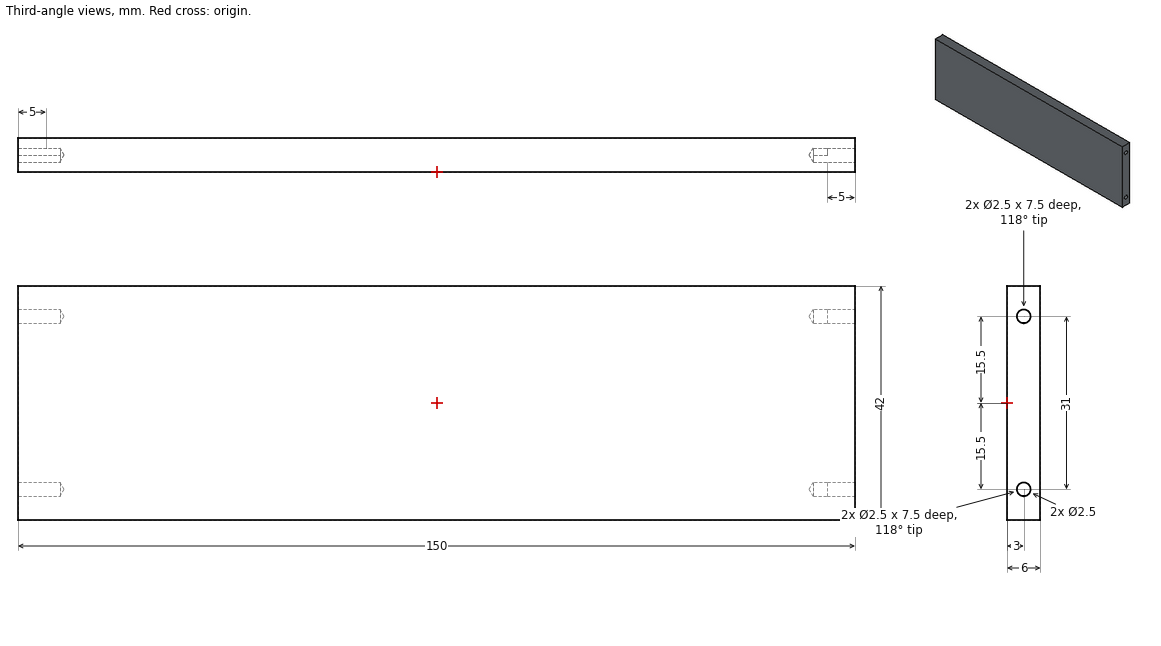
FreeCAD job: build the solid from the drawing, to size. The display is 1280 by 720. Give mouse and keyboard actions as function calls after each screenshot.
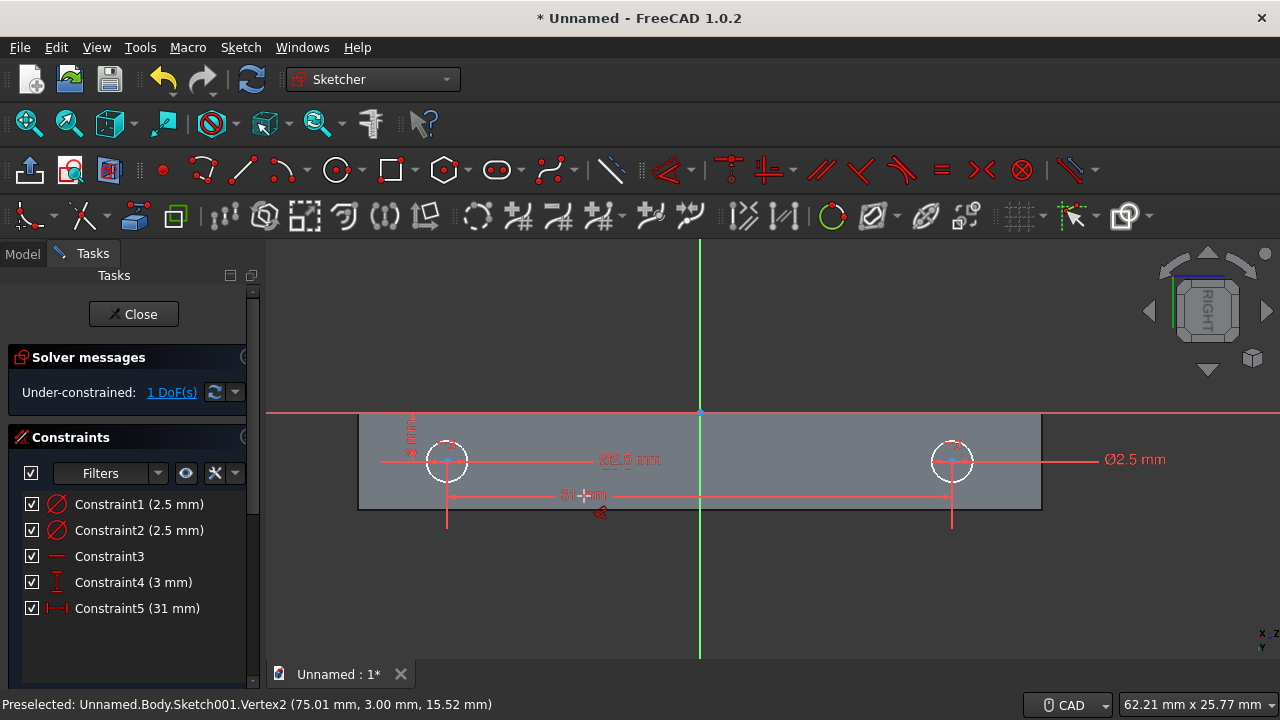
click(447, 462)
click(574, 379)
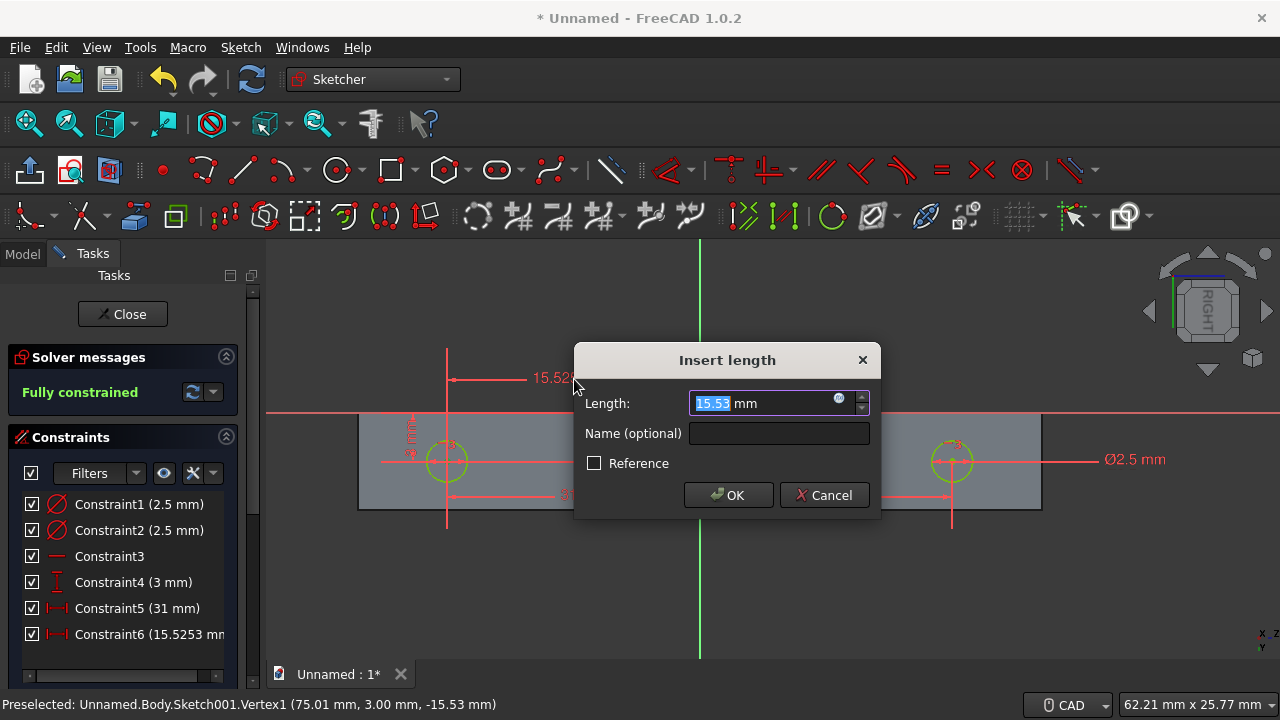
text(15.5)
key(Return)
key(Escape)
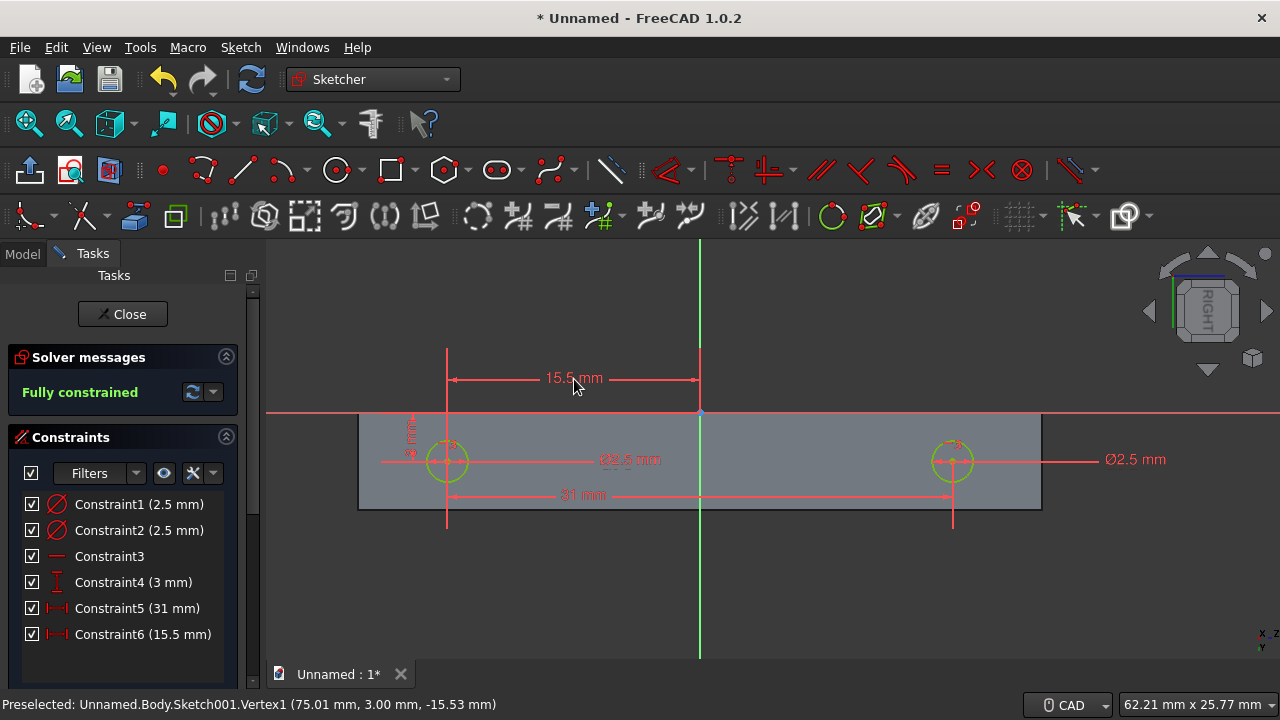
click(123, 314)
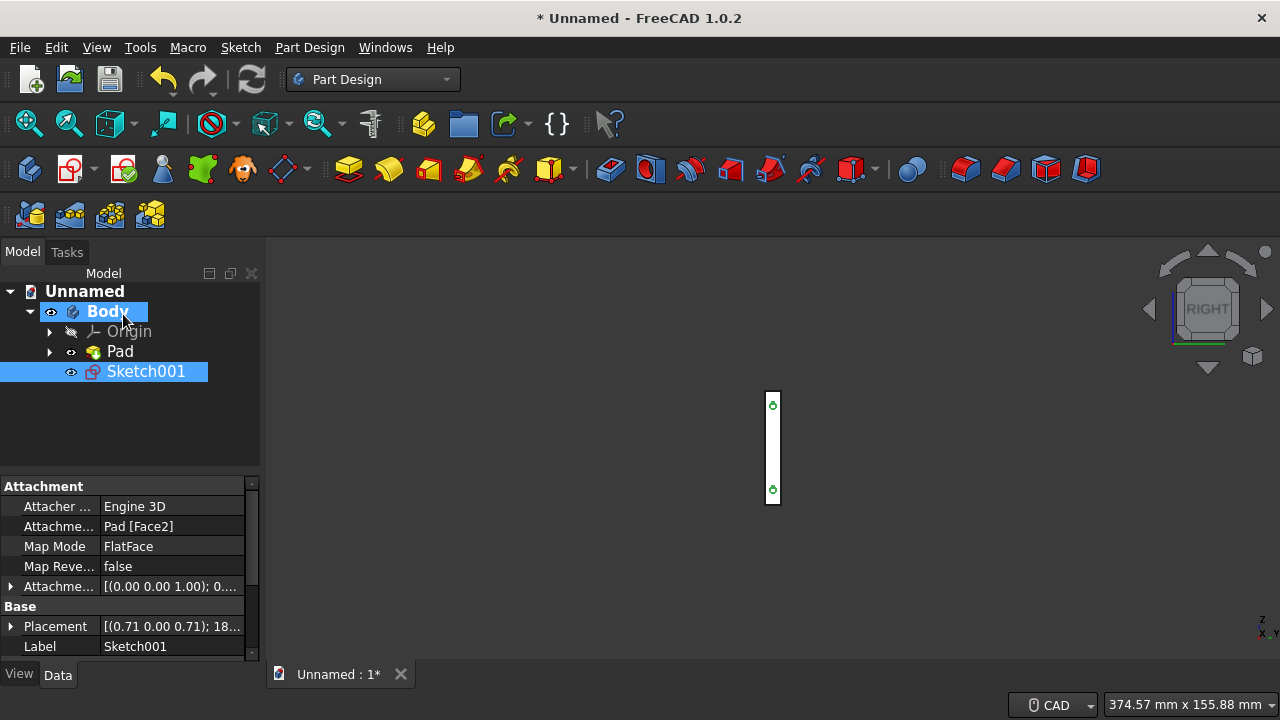
click(612, 170)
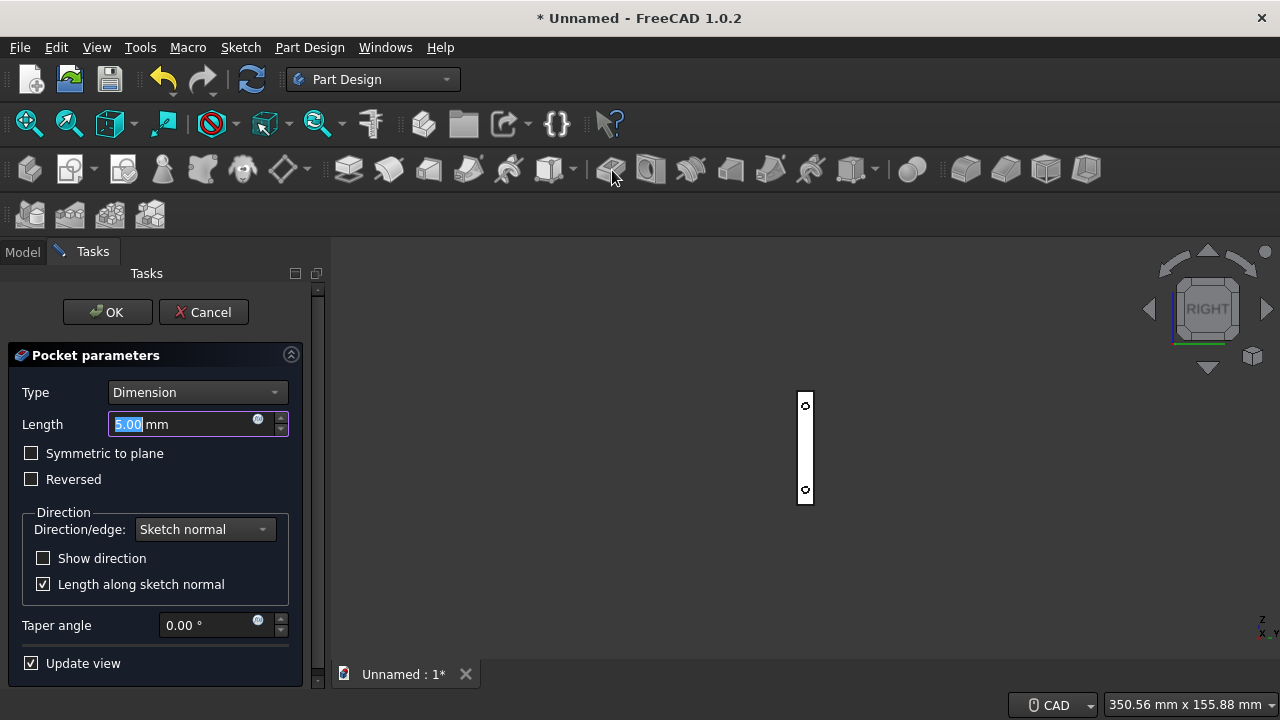
text(5)
key(Tab)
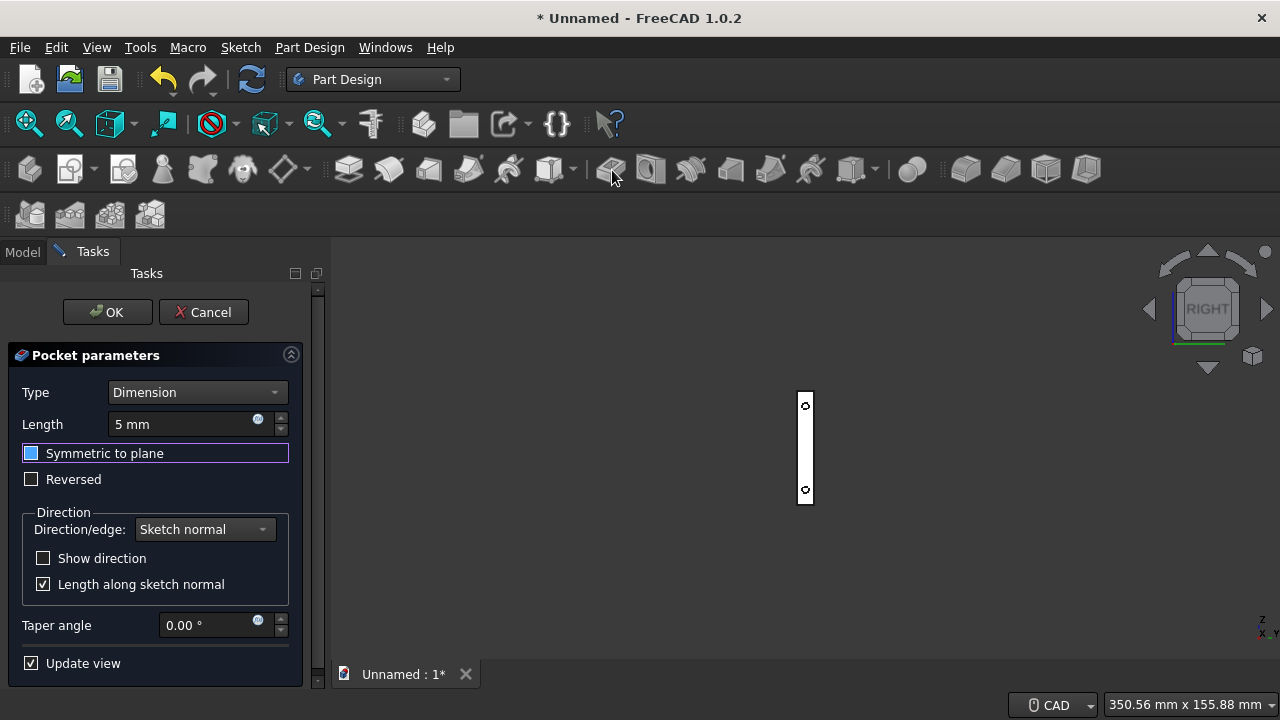
click(108, 312)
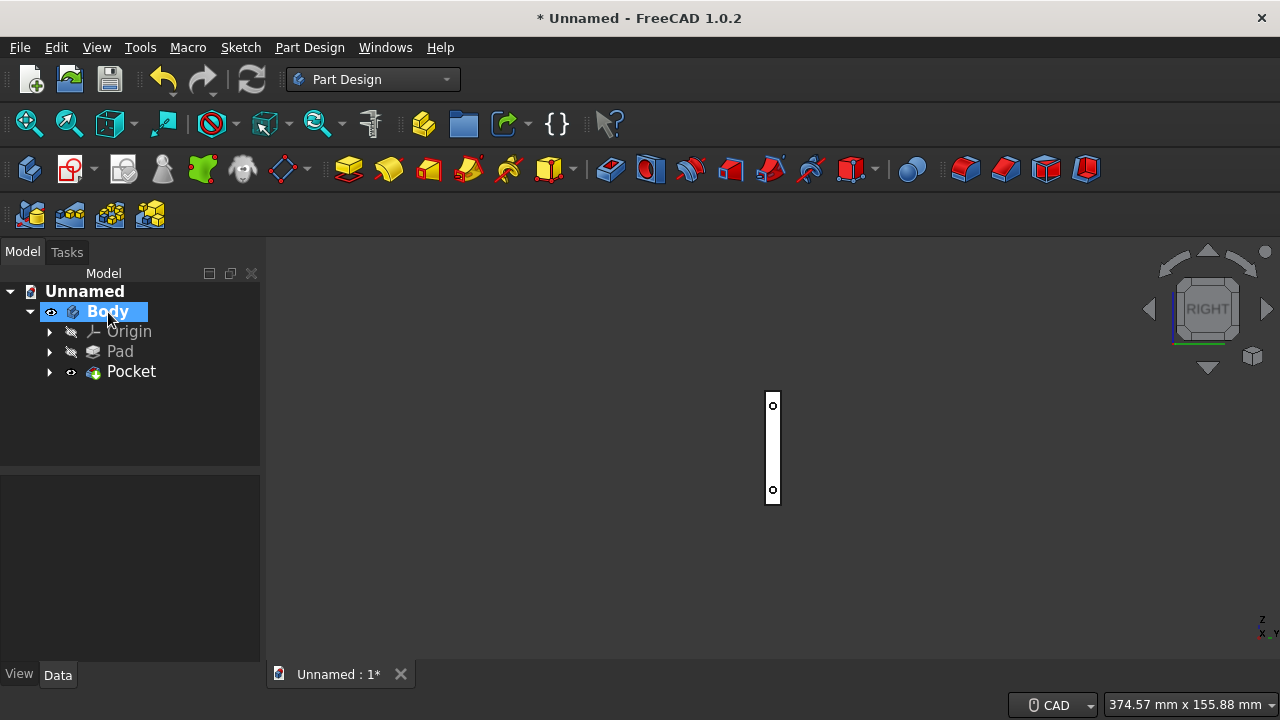
click(30, 124)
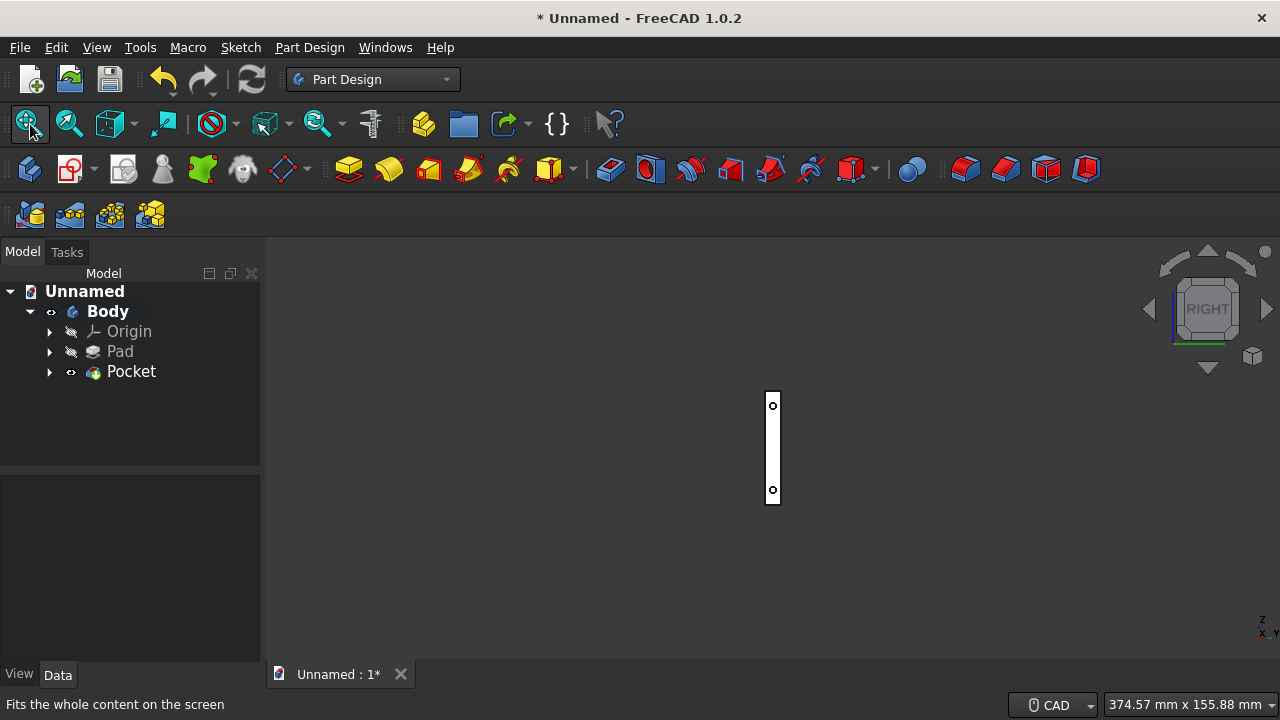
click(50, 332)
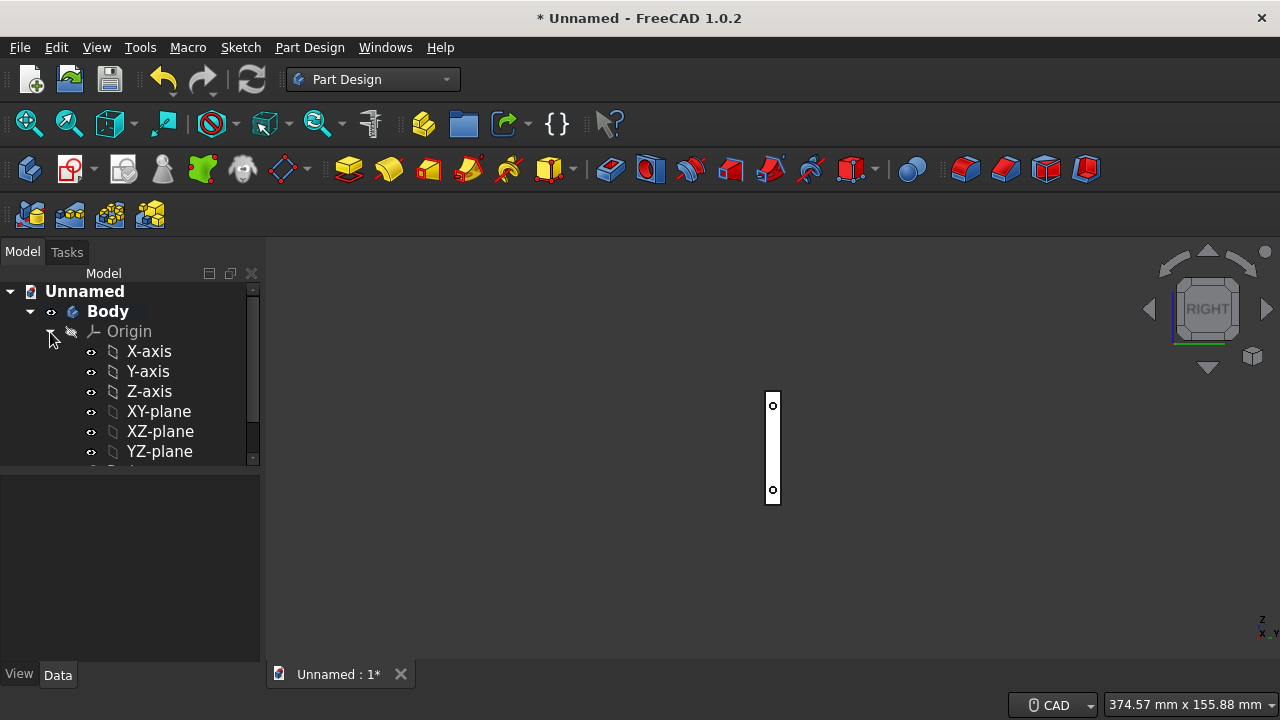
click(136, 452)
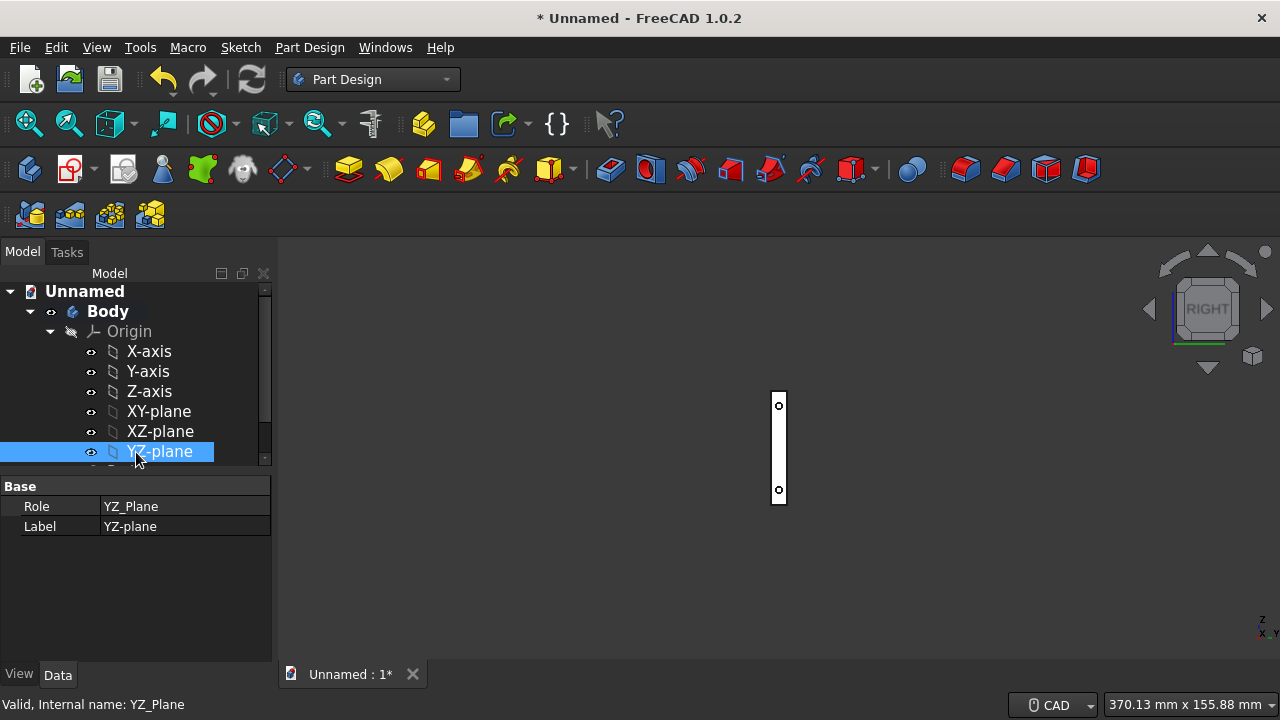
click(284, 170)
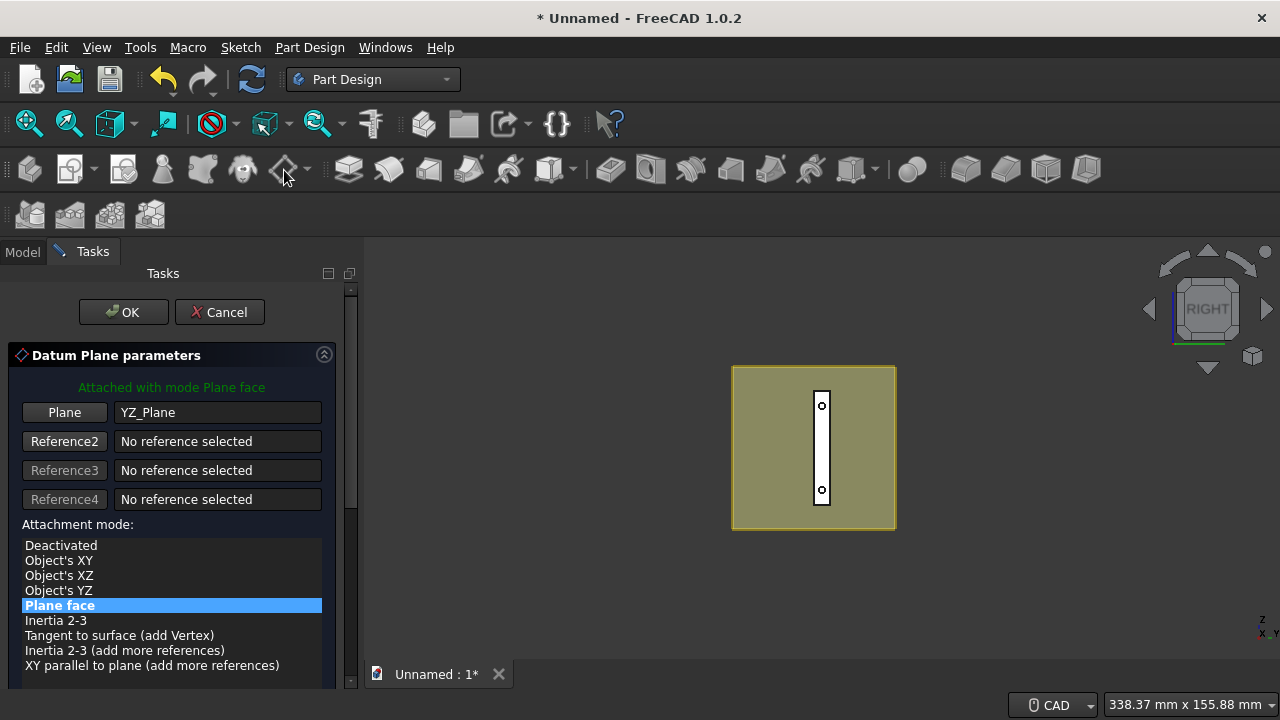
scroll(351, 486, down, 4)